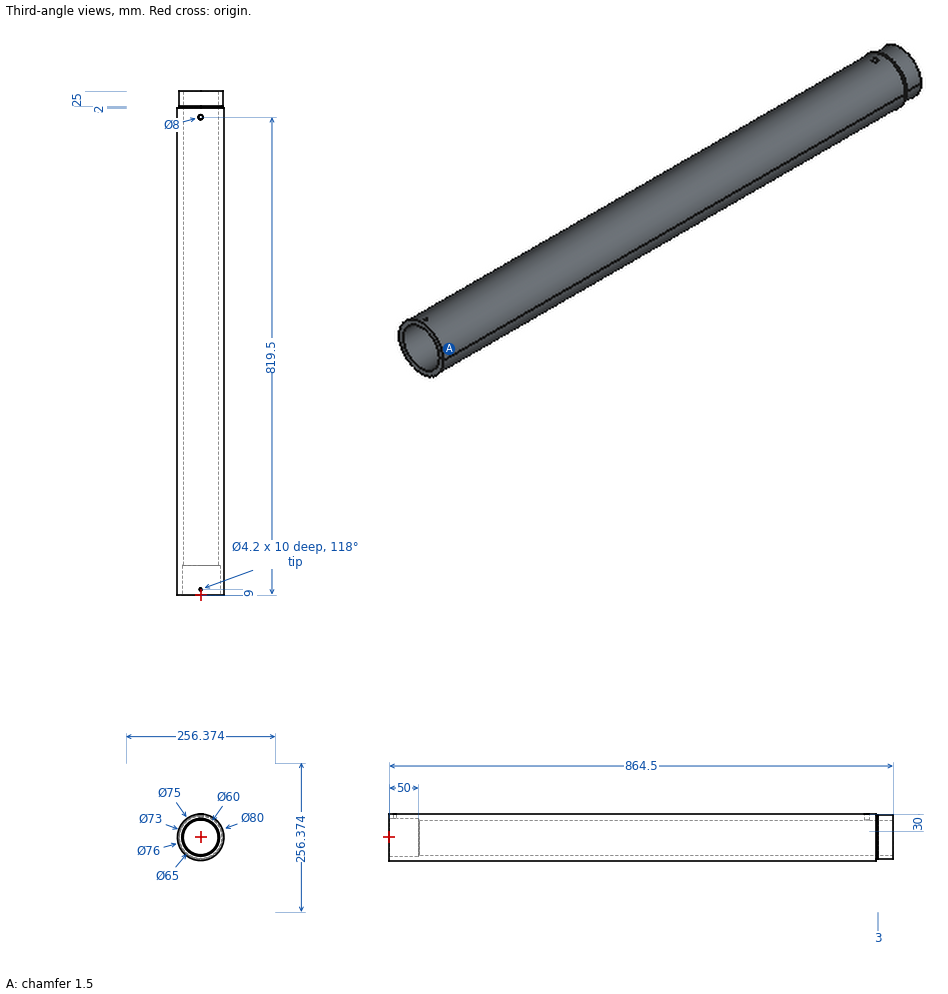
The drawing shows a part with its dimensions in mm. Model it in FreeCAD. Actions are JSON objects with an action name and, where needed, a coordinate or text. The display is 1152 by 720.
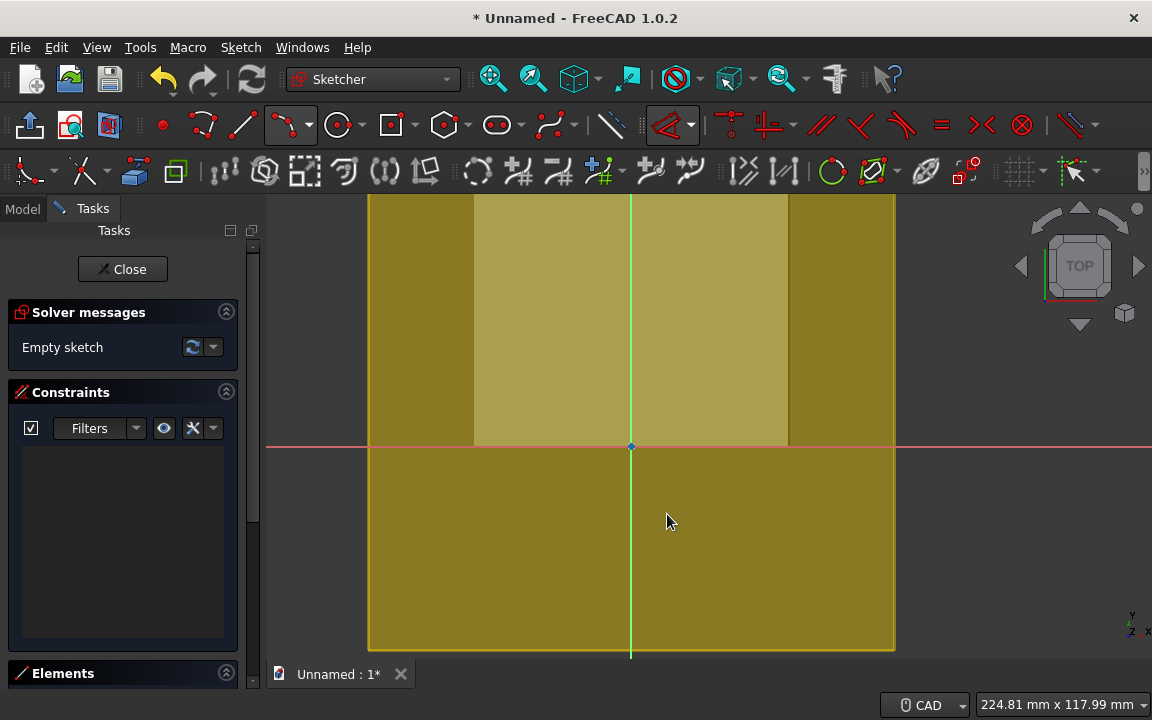
{"action": "scroll", "coordinate": [631, 410], "scroll_direction": "up", "scroll_amount": 14}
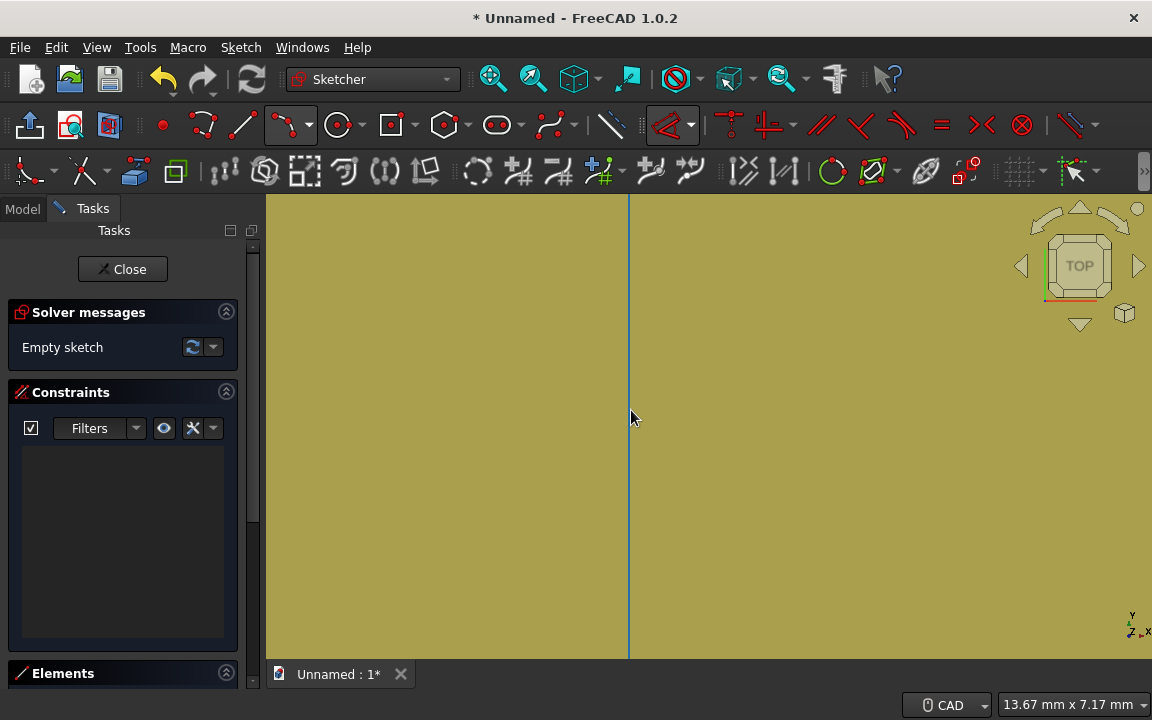
{"action": "key", "text": "g c"}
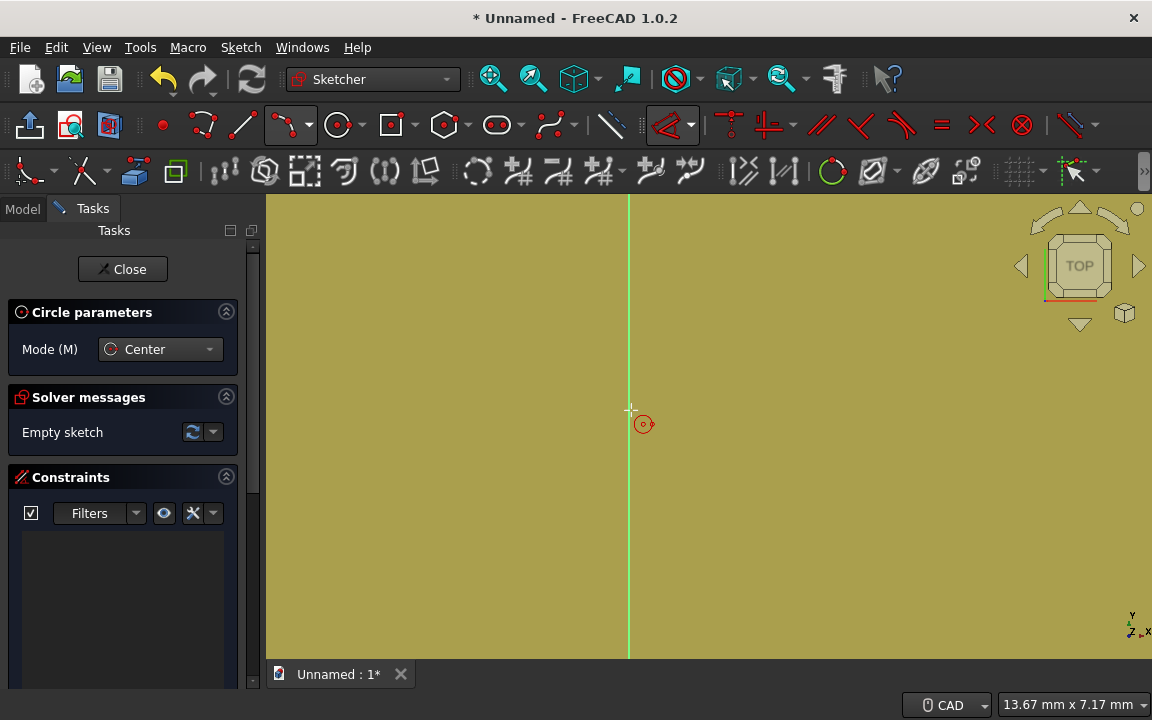
{"action": "left_click", "coordinate": [629, 426]}
{"action": "mouse_move", "coordinate": [725, 330]}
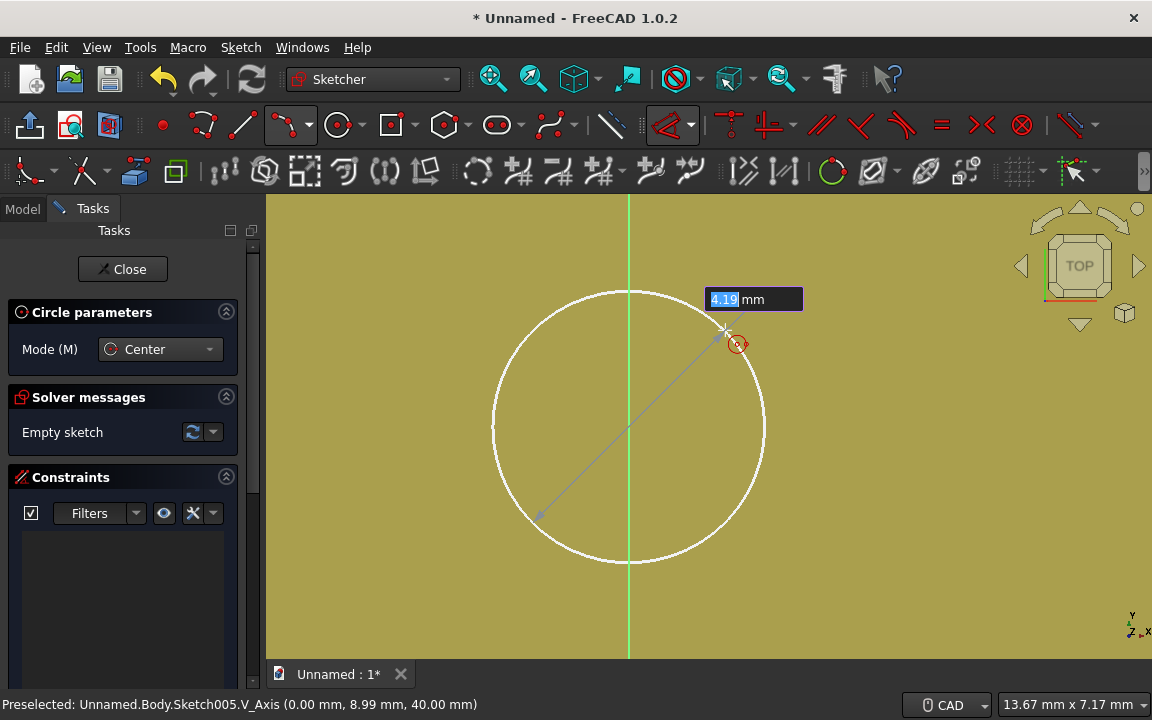
{"action": "type", "text": "4.2"}
{"action": "key", "text": "Return"}
{"action": "key", "text": "Escape"}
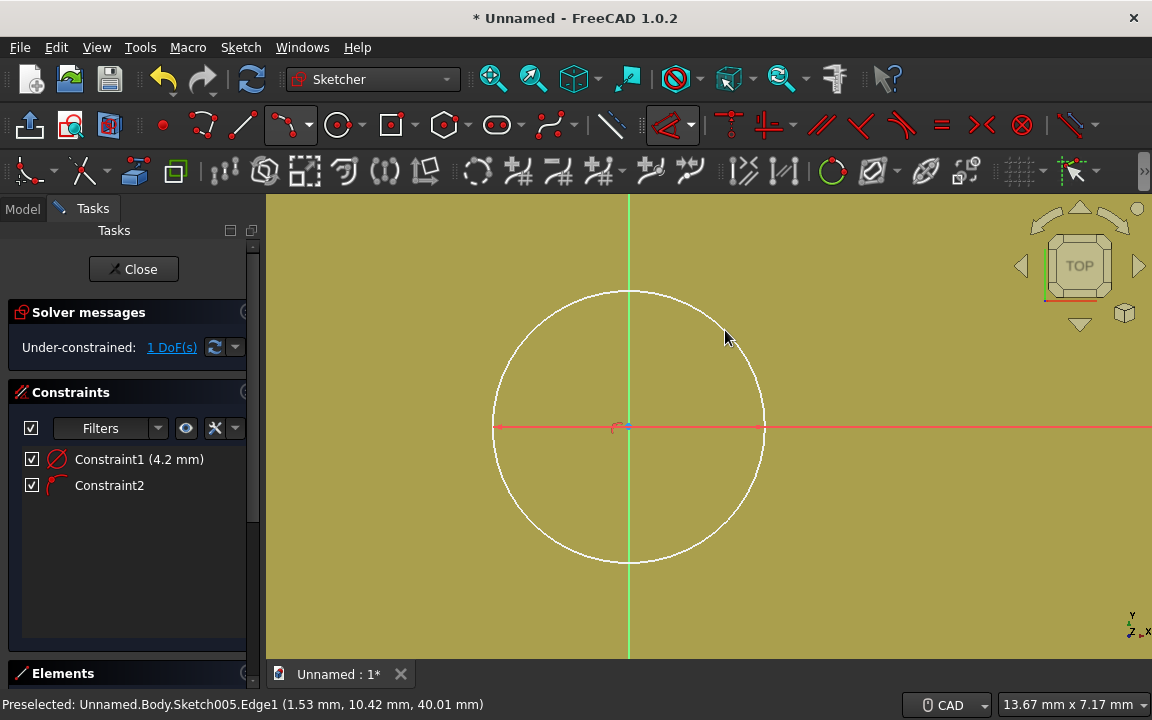
{"action": "left_click", "coordinate": [666, 126]}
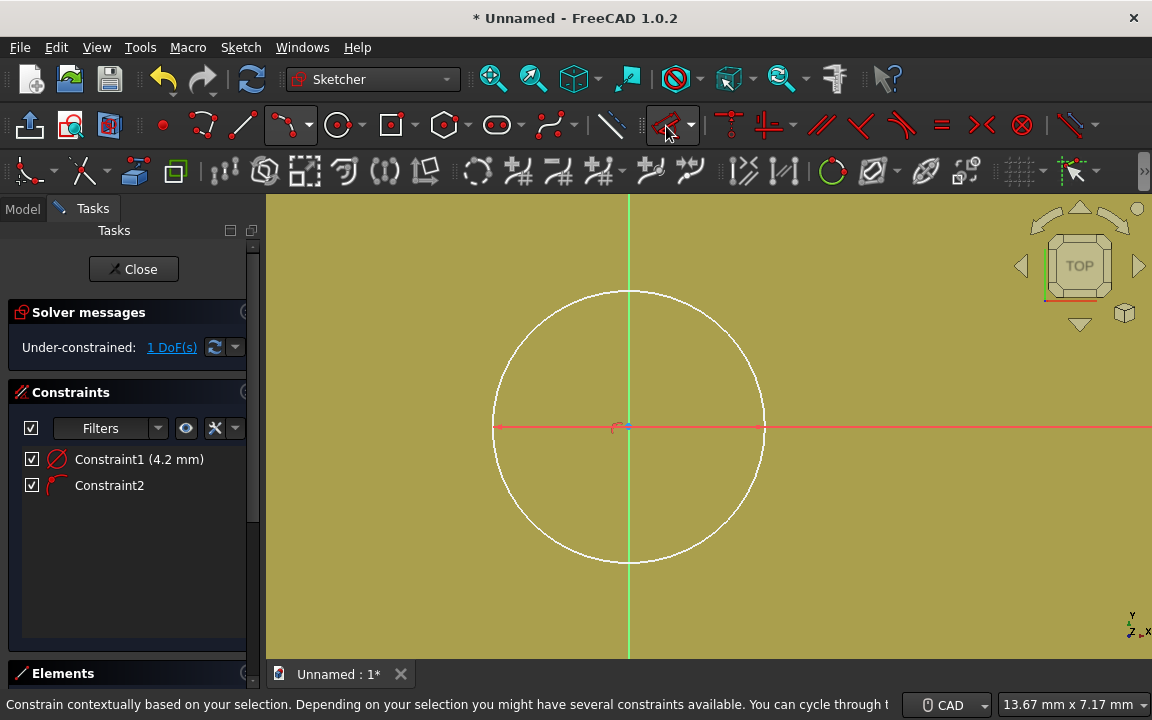
{"action": "left_click", "coordinate": [629, 427]}
{"action": "left_click", "coordinate": [663, 529]}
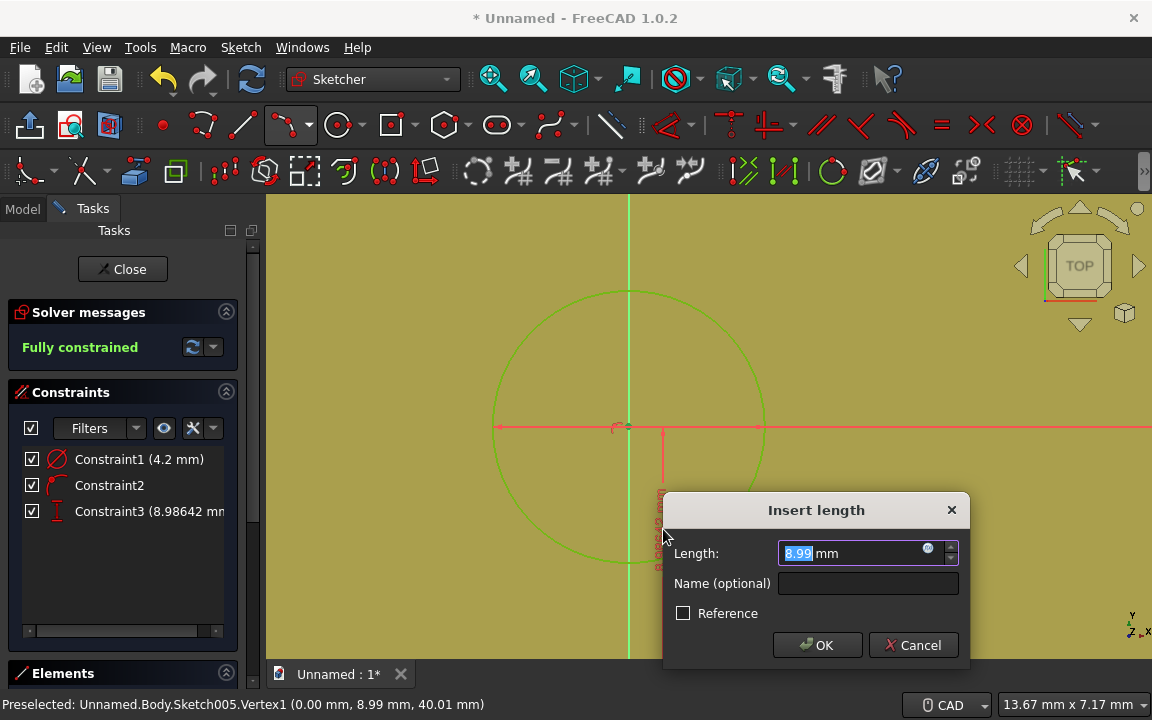
{"action": "type", "text": "9"}
{"action": "key", "text": "Return"}
{"action": "key", "text": "Escape"}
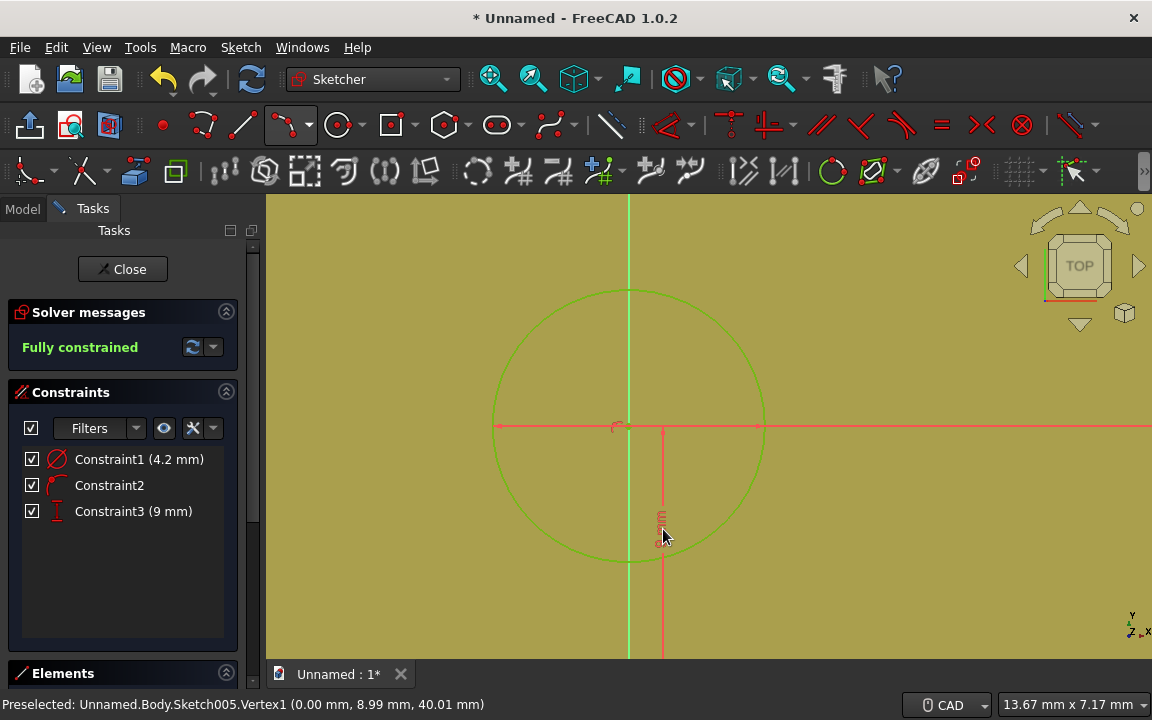
{"action": "left_click", "coordinate": [123, 269]}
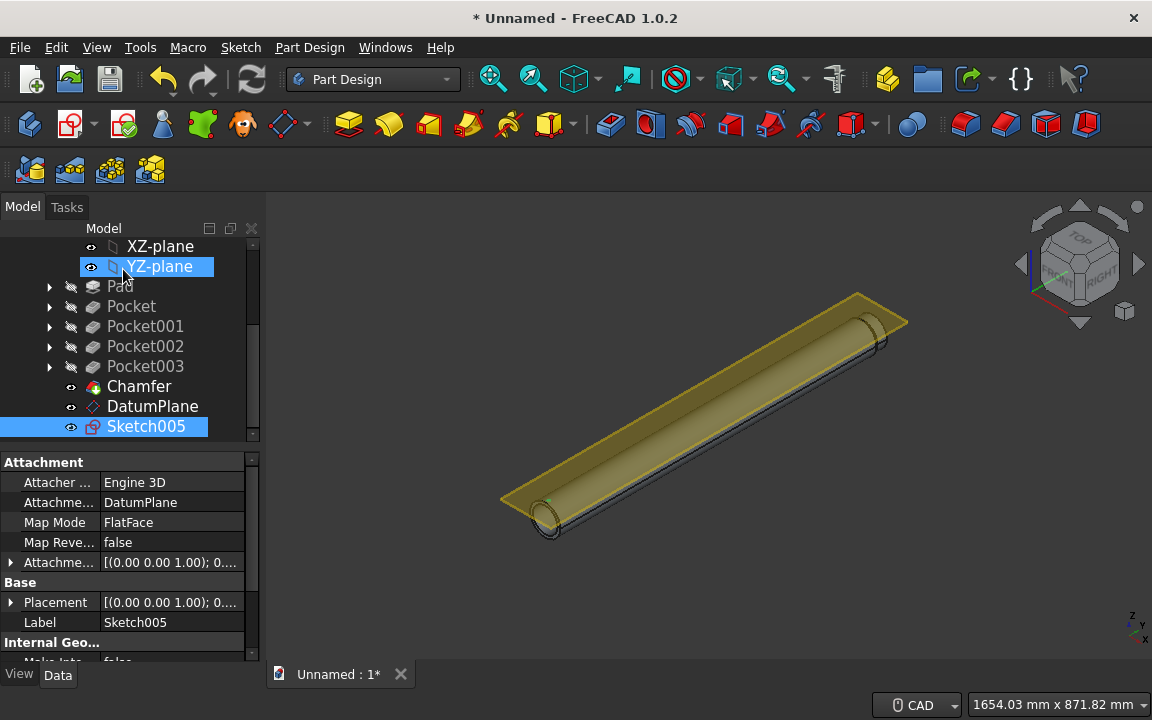
{"action": "left_click", "coordinate": [652, 124]}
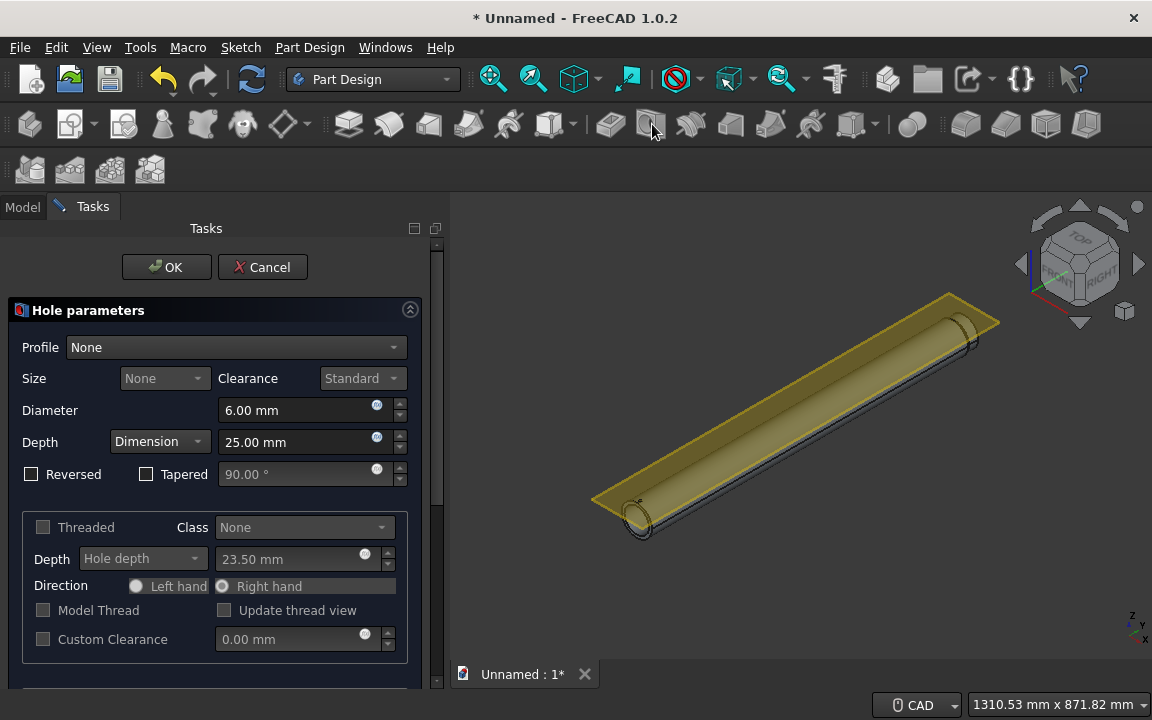
{"action": "triple_click", "coordinate": [305, 410]}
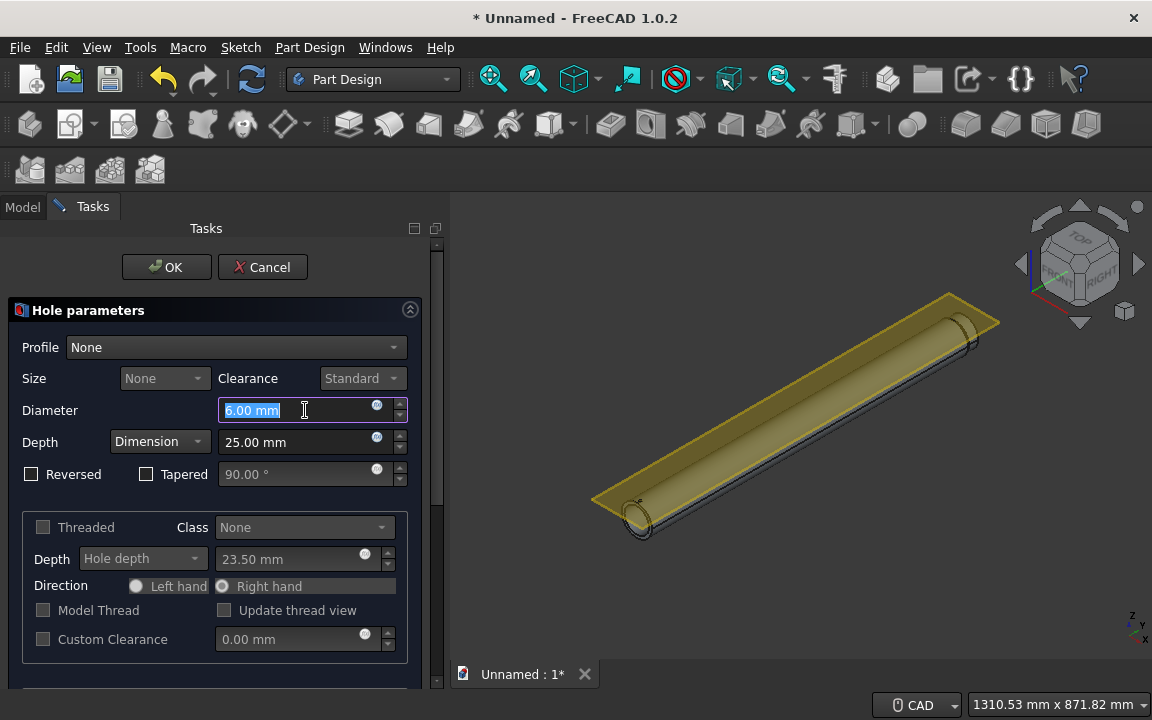
{"action": "type", "text": "4.2"}
{"action": "key", "text": "Tab"}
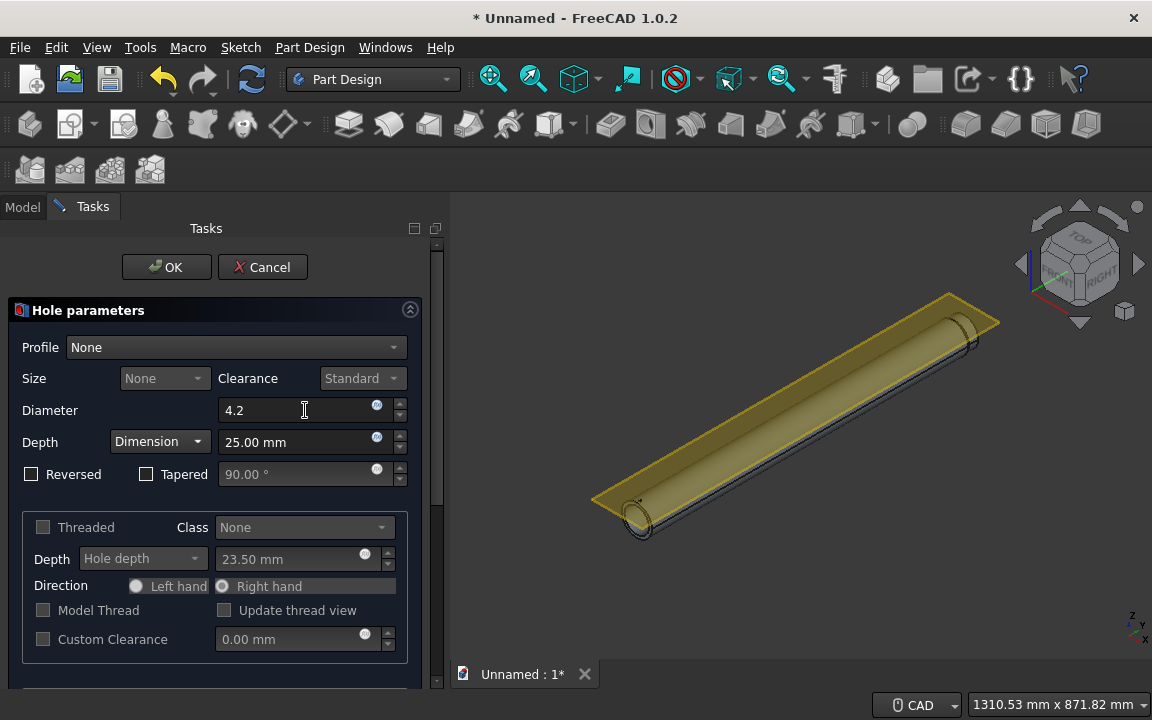
{"action": "triple_click", "coordinate": [305, 442]}